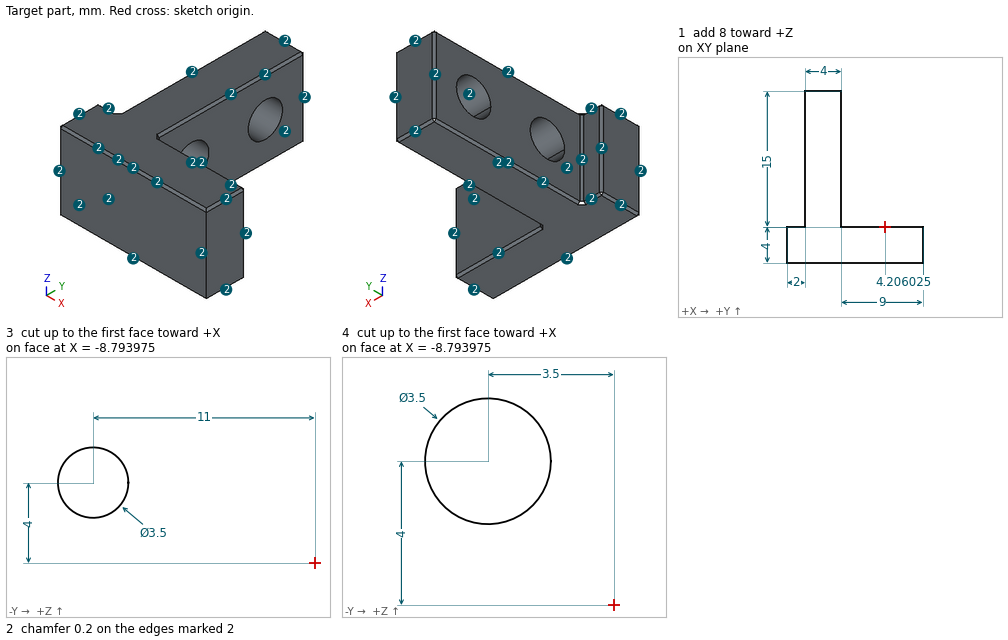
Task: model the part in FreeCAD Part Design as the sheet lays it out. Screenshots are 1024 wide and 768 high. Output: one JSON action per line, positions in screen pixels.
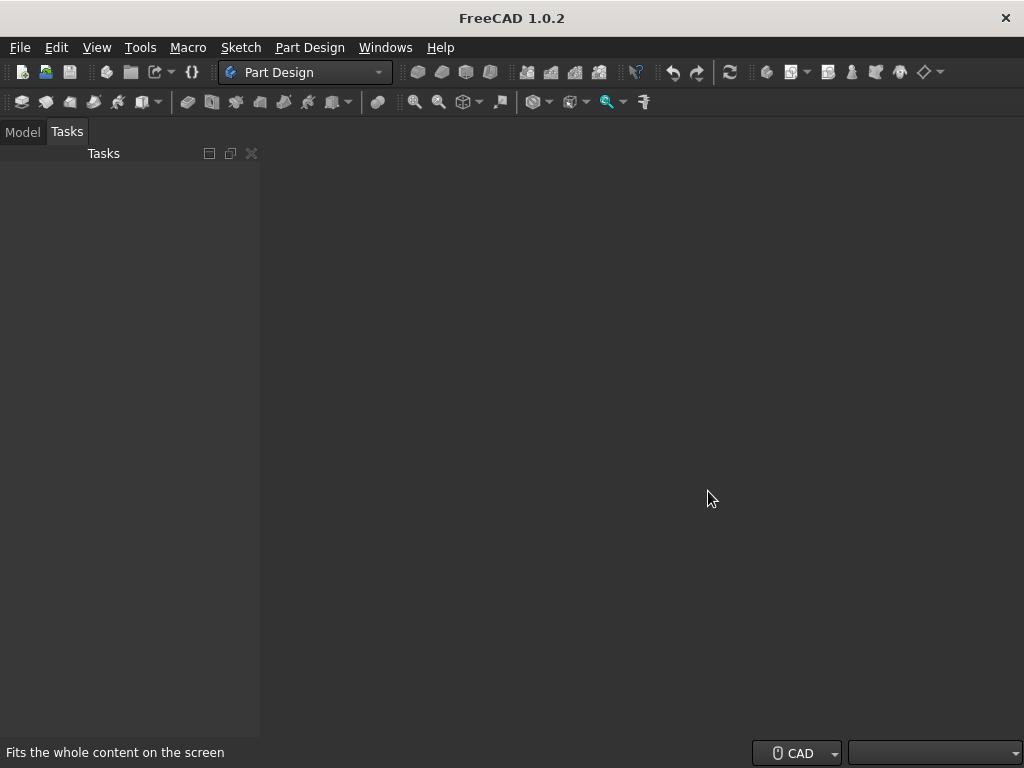
{"action": "left_click", "coordinate": [22, 72]}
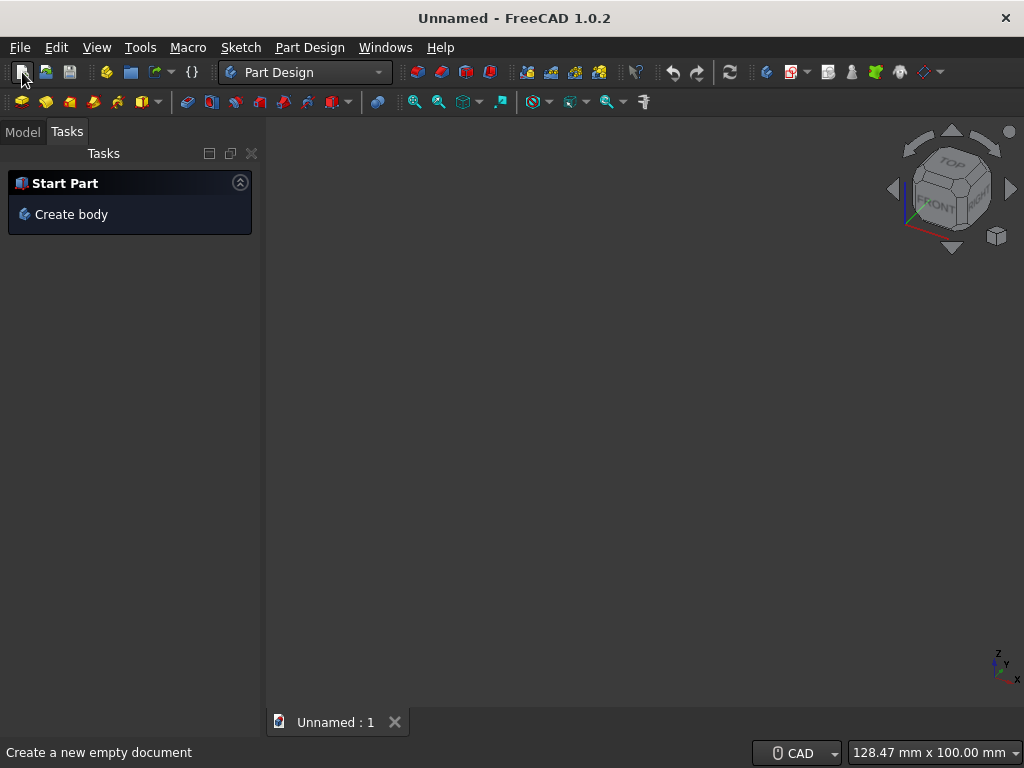
{"action": "left_click", "coordinate": [792, 72]}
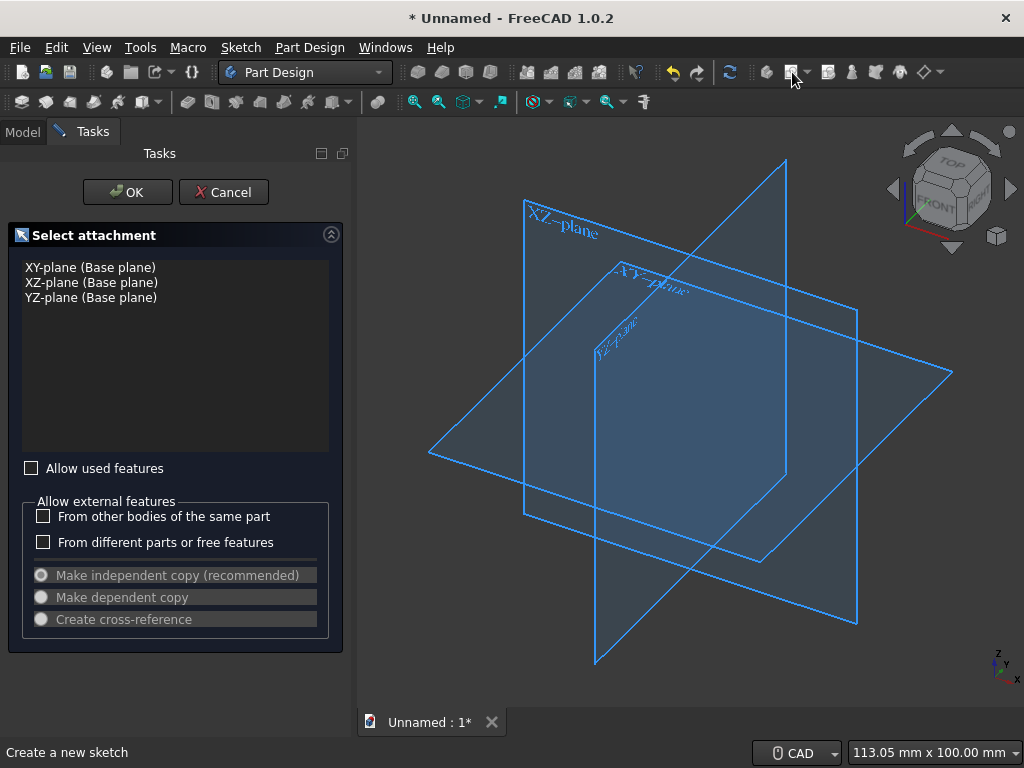
{"action": "left_click", "coordinate": [82, 268]}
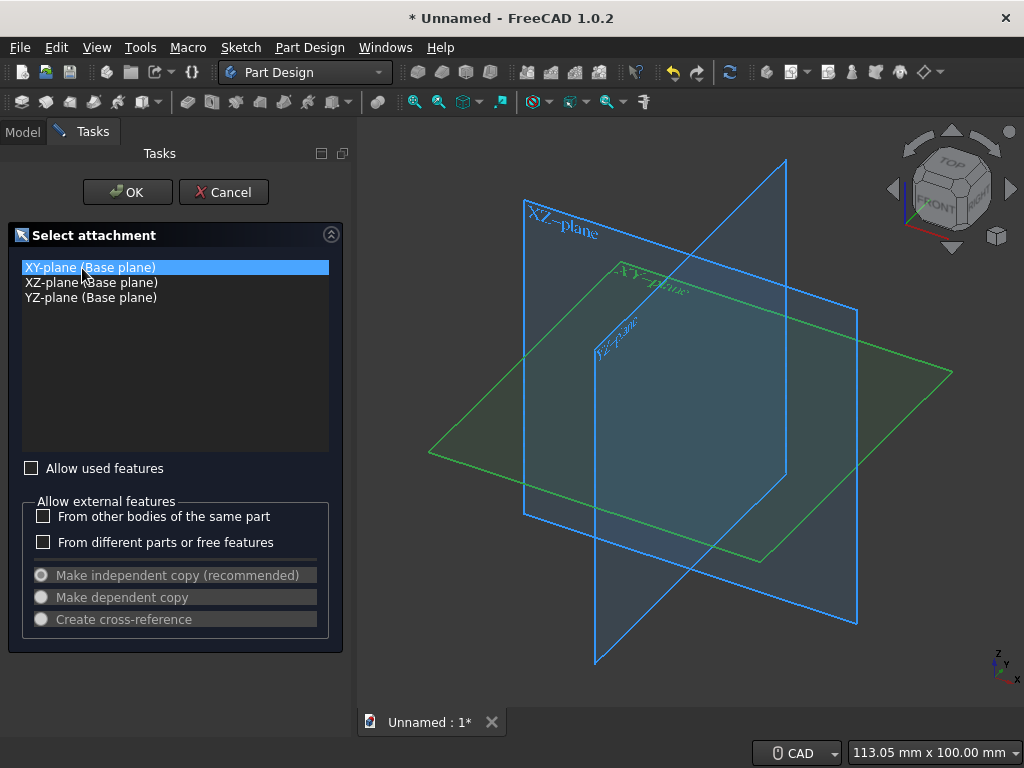
{"action": "left_click", "coordinate": [128, 192]}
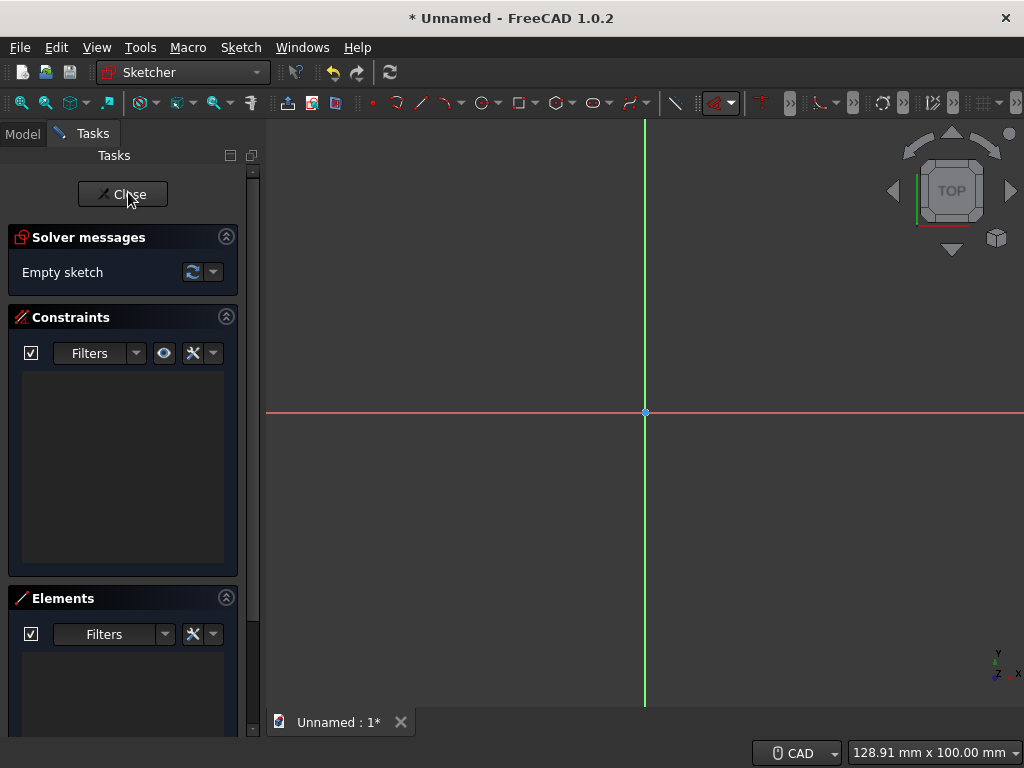
{"action": "scroll", "coordinate": [647, 367], "scroll_direction": "up", "scroll_amount": 6}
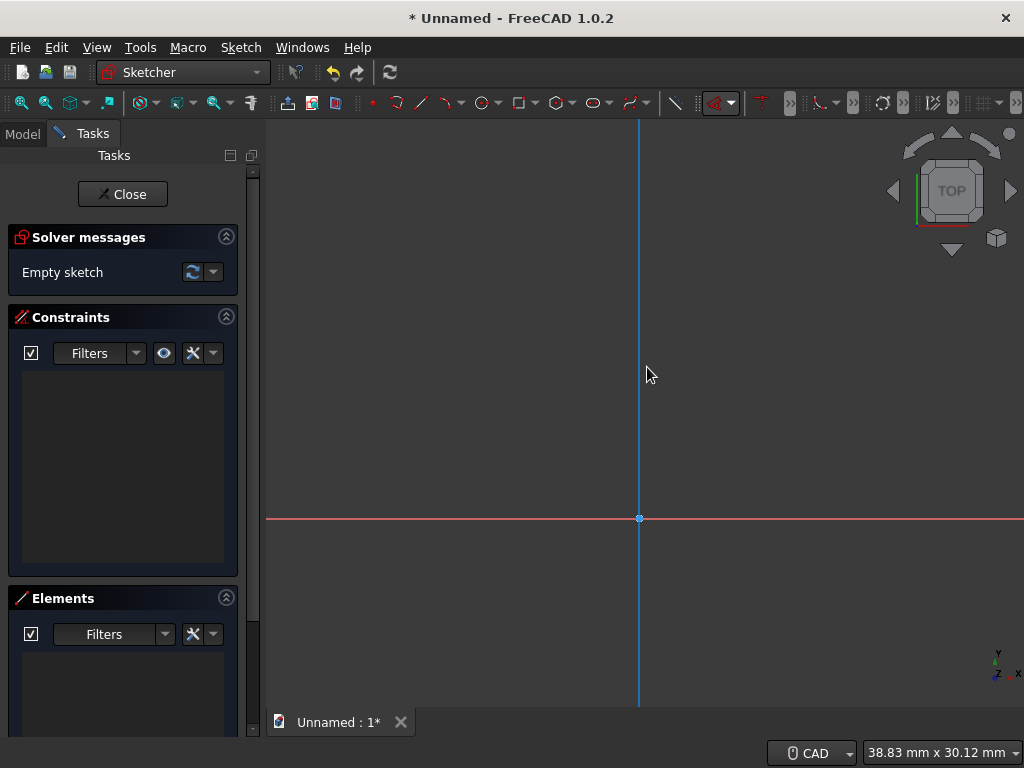
{"action": "left_click", "coordinate": [398, 104]}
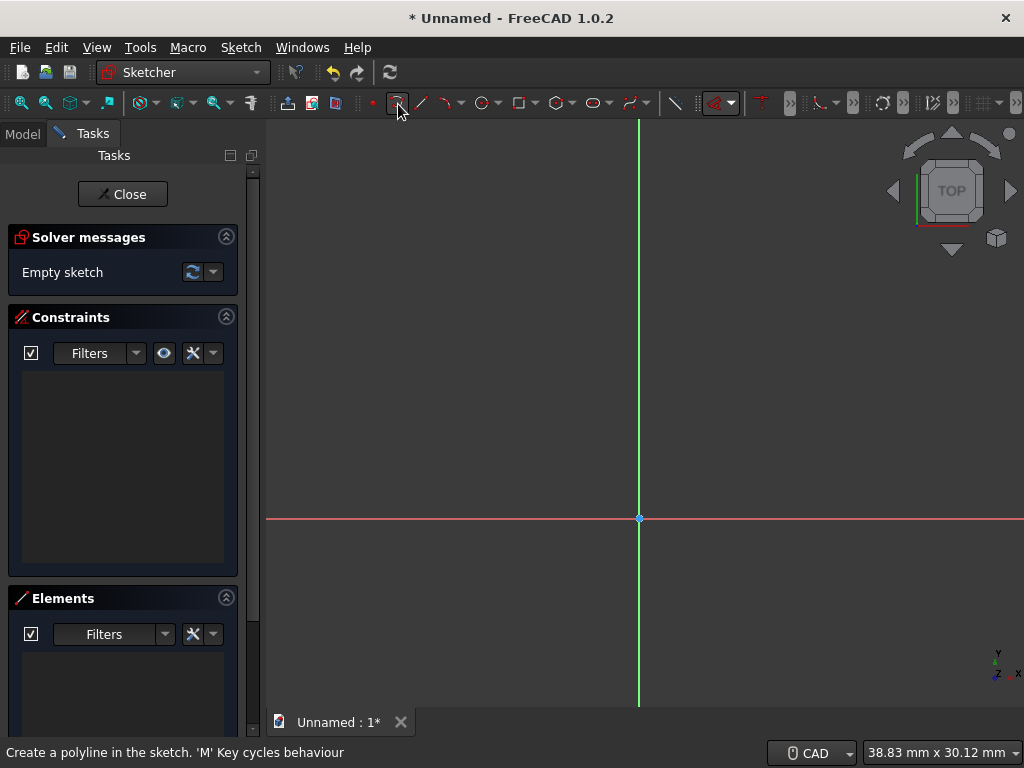
{"action": "left_click", "coordinate": [721, 519]}
{"action": "left_click", "coordinate": [546, 510]}
{"action": "left_click", "coordinate": [546, 226]}
{"action": "left_click", "coordinate": [468, 226]}
{"action": "left_click", "coordinate": [468, 519]}
{"action": "left_click", "coordinate": [428, 510]}
{"action": "left_click", "coordinate": [428, 597]}
{"action": "left_click", "coordinate": [721, 597]}
{"action": "left_click", "coordinate": [721, 519]}
{"action": "key", "text": "Escape"}
{"action": "key", "text": "Escape"}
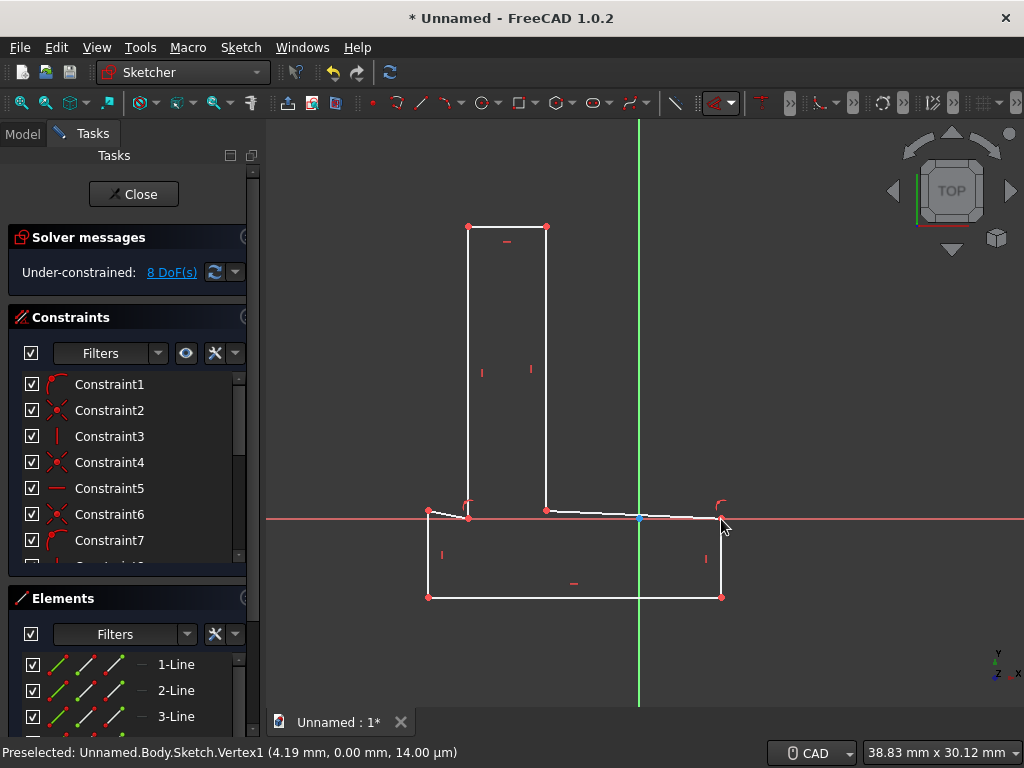
{"action": "left_click", "coordinate": [668, 516]}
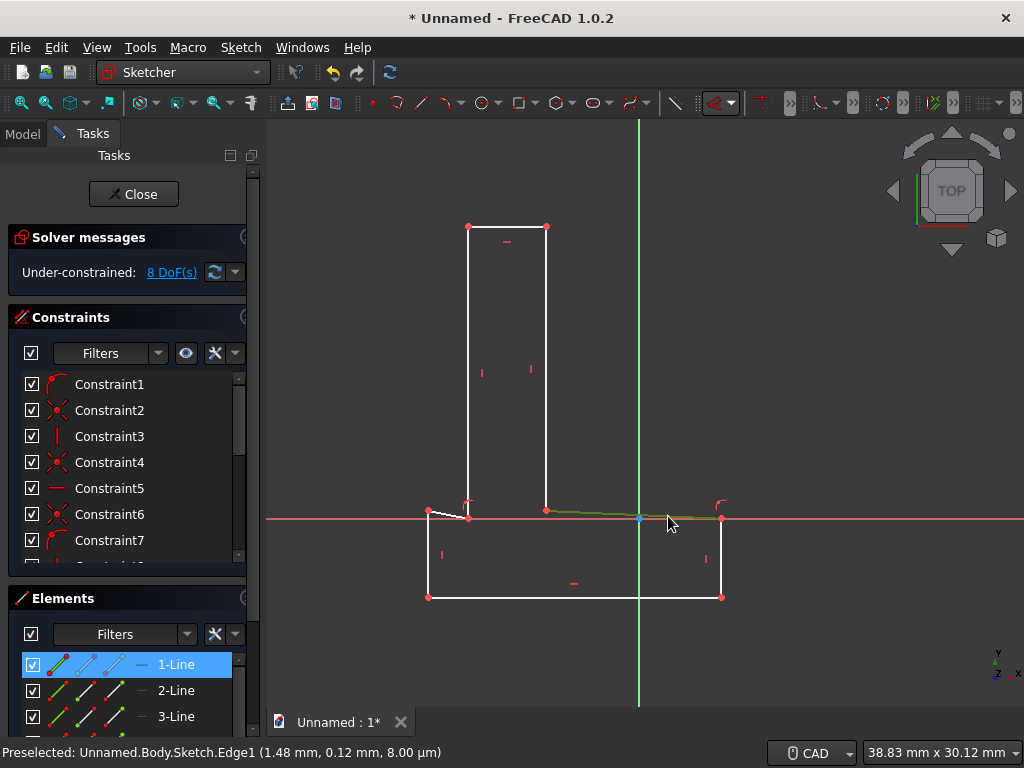
{"action": "key", "text": "h"}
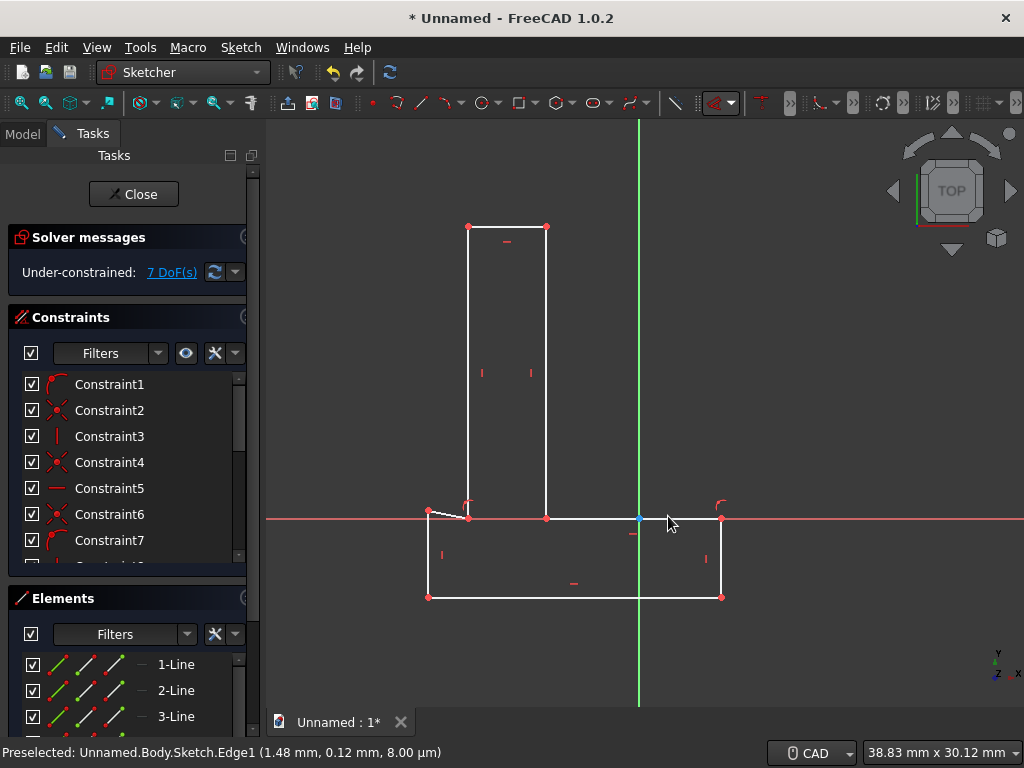
{"action": "left_click", "coordinate": [456, 516]}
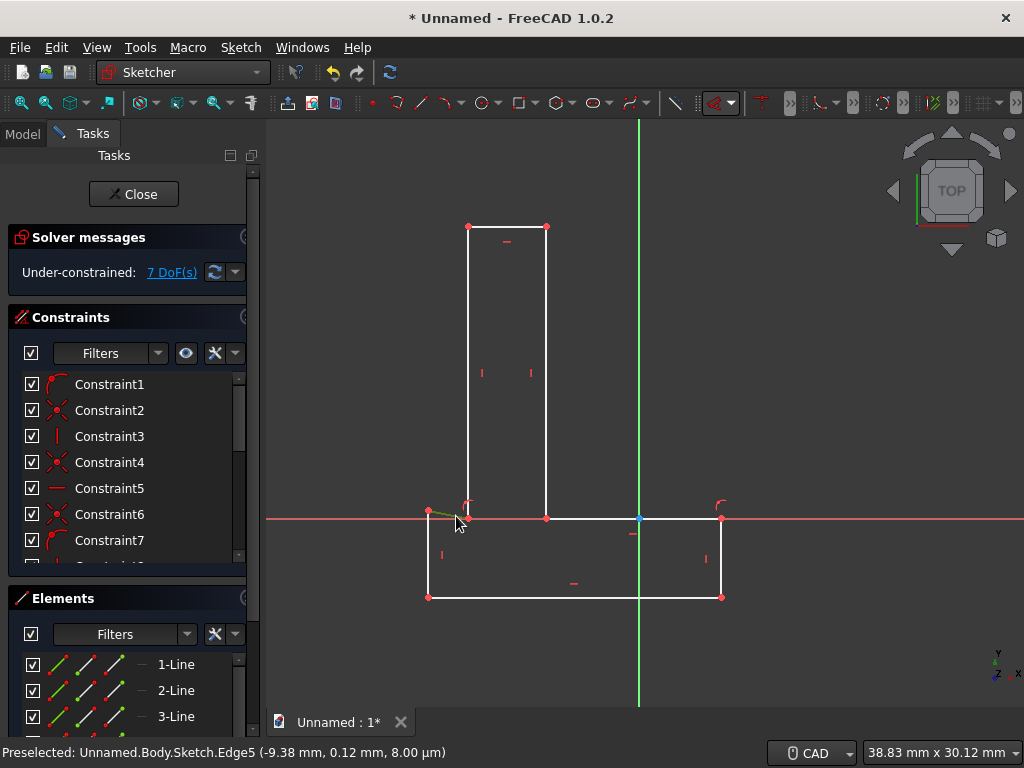
{"action": "key", "text": "h"}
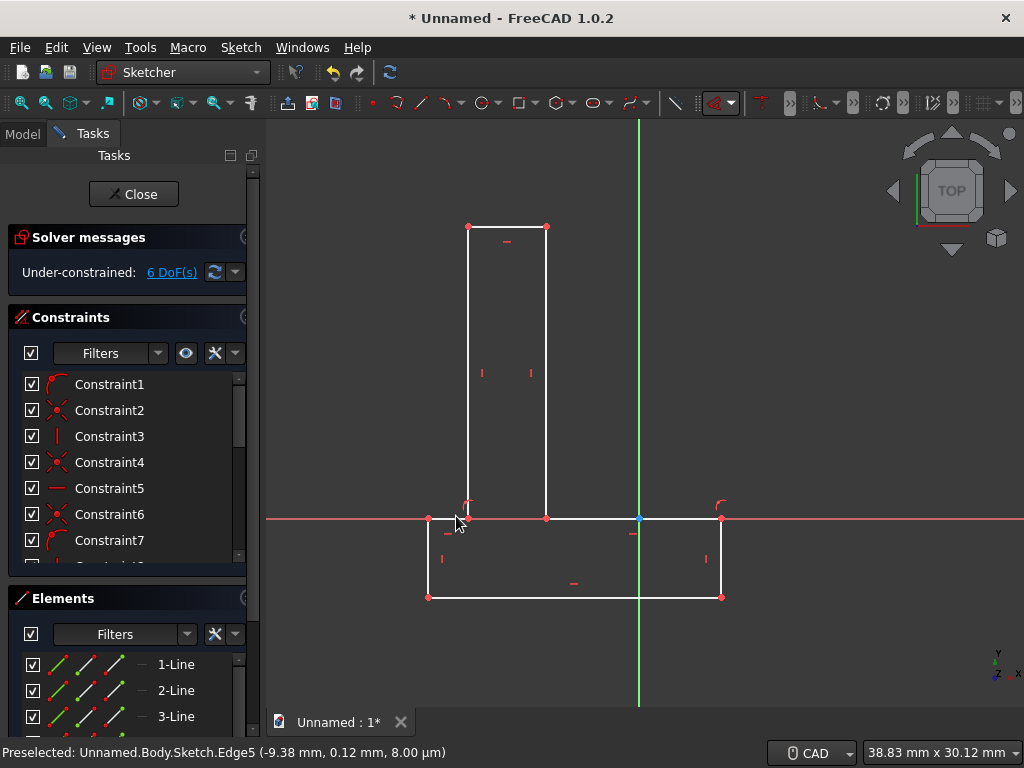
{"action": "left_click", "coordinate": [668, 519]}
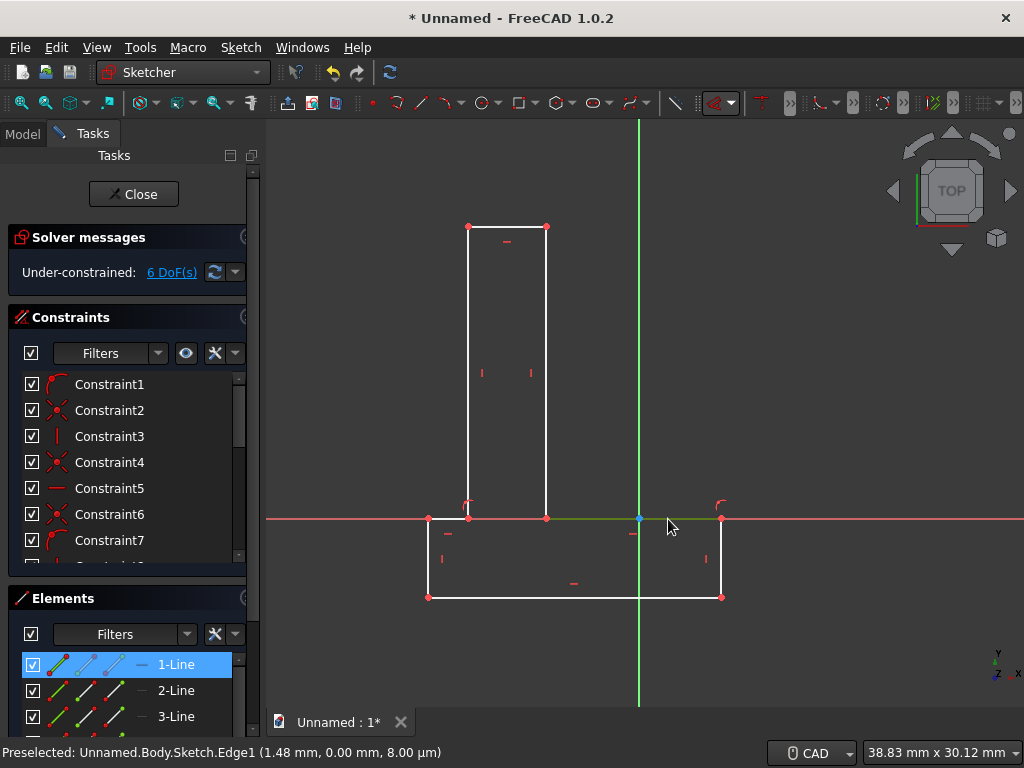
{"action": "key", "text": "l"}